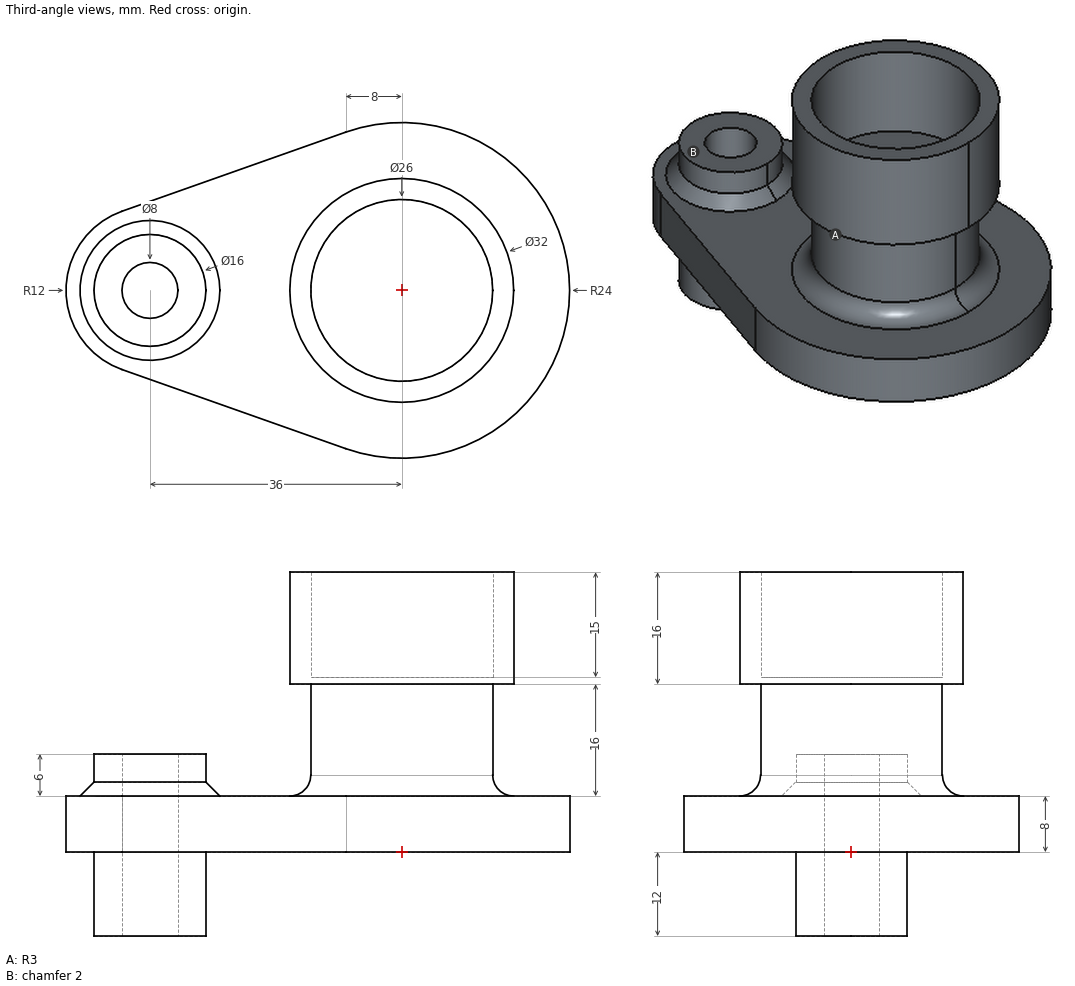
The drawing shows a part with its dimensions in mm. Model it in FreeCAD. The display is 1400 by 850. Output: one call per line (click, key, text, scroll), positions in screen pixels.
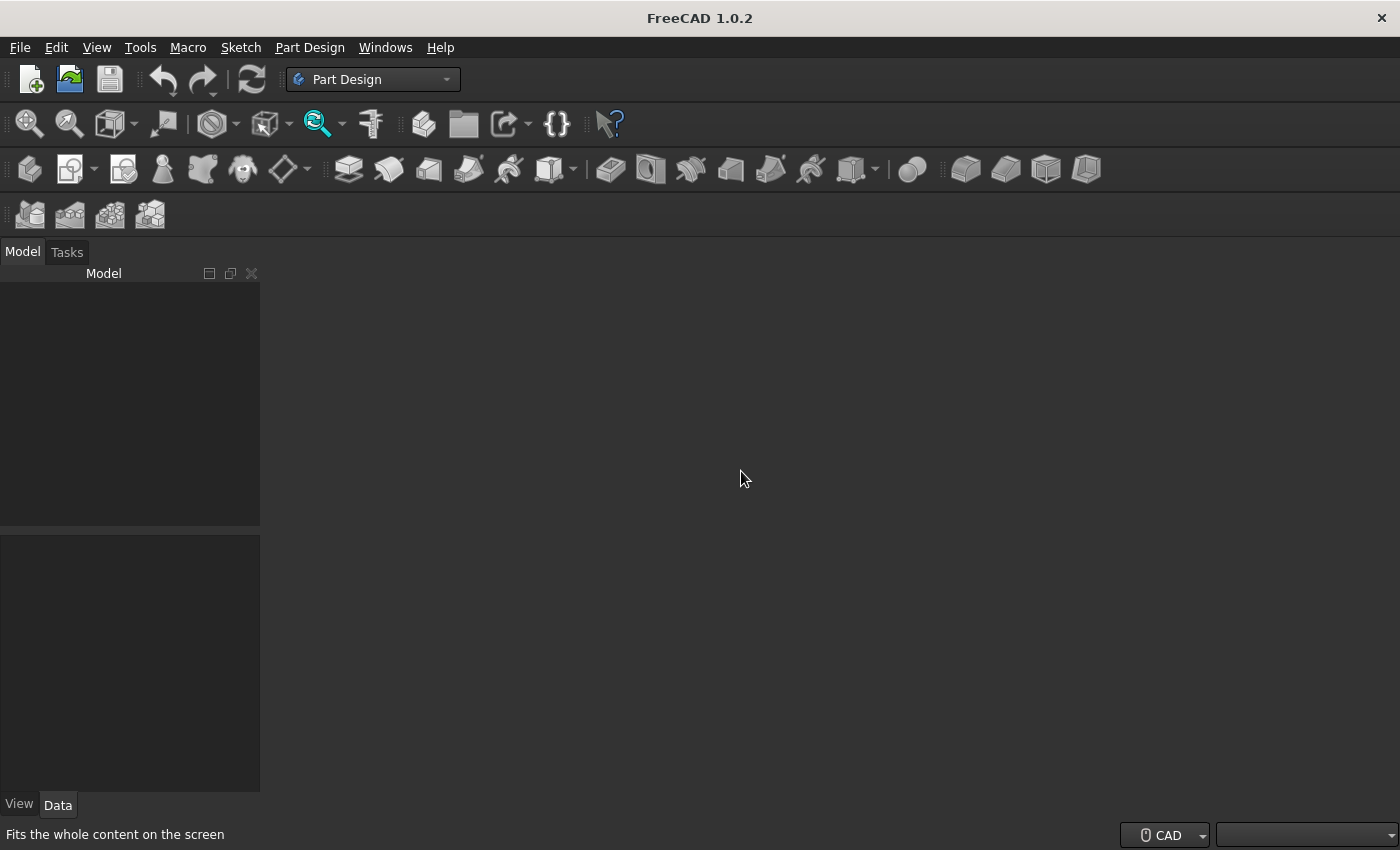
key(ctrl+n)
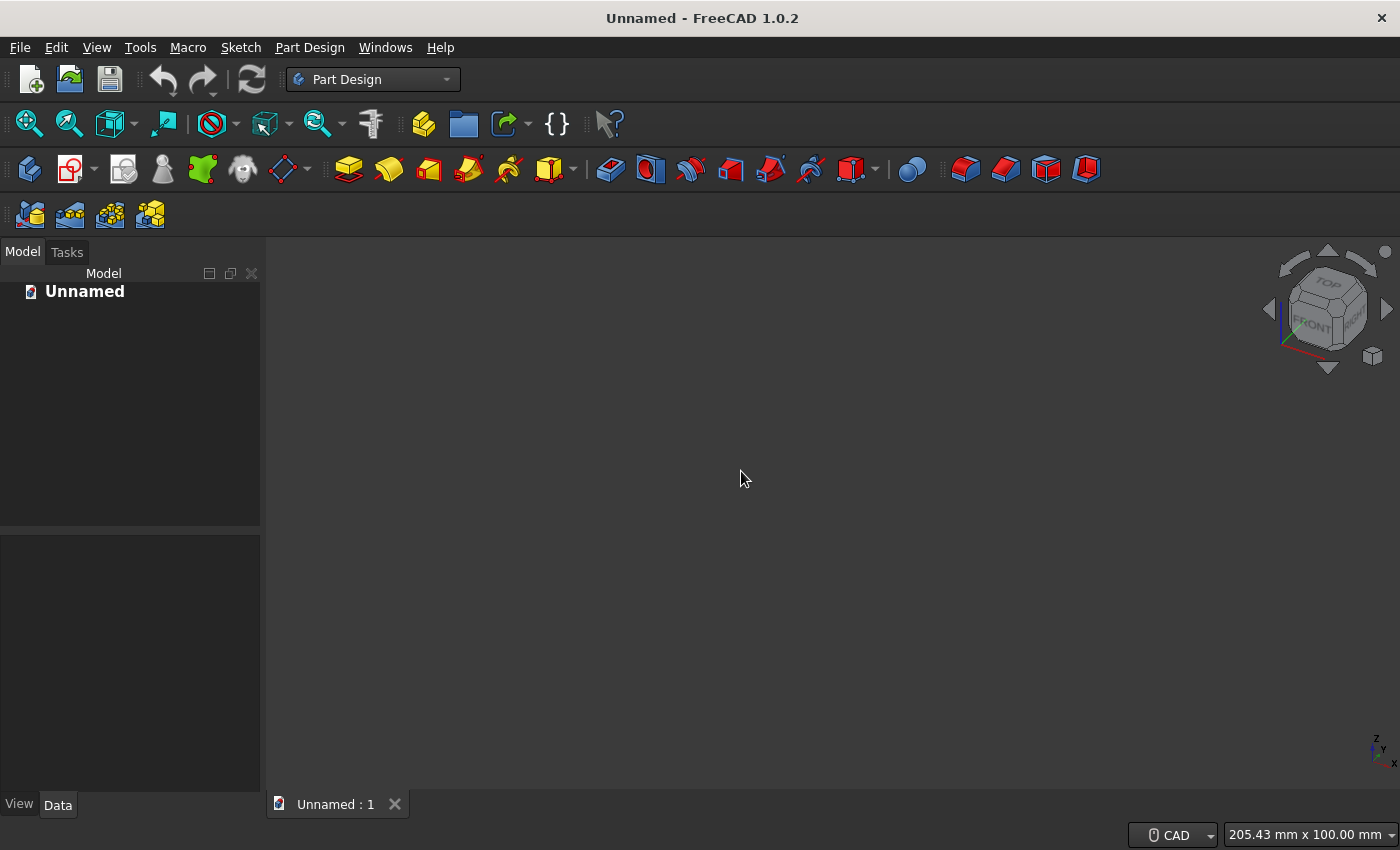
click(70, 170)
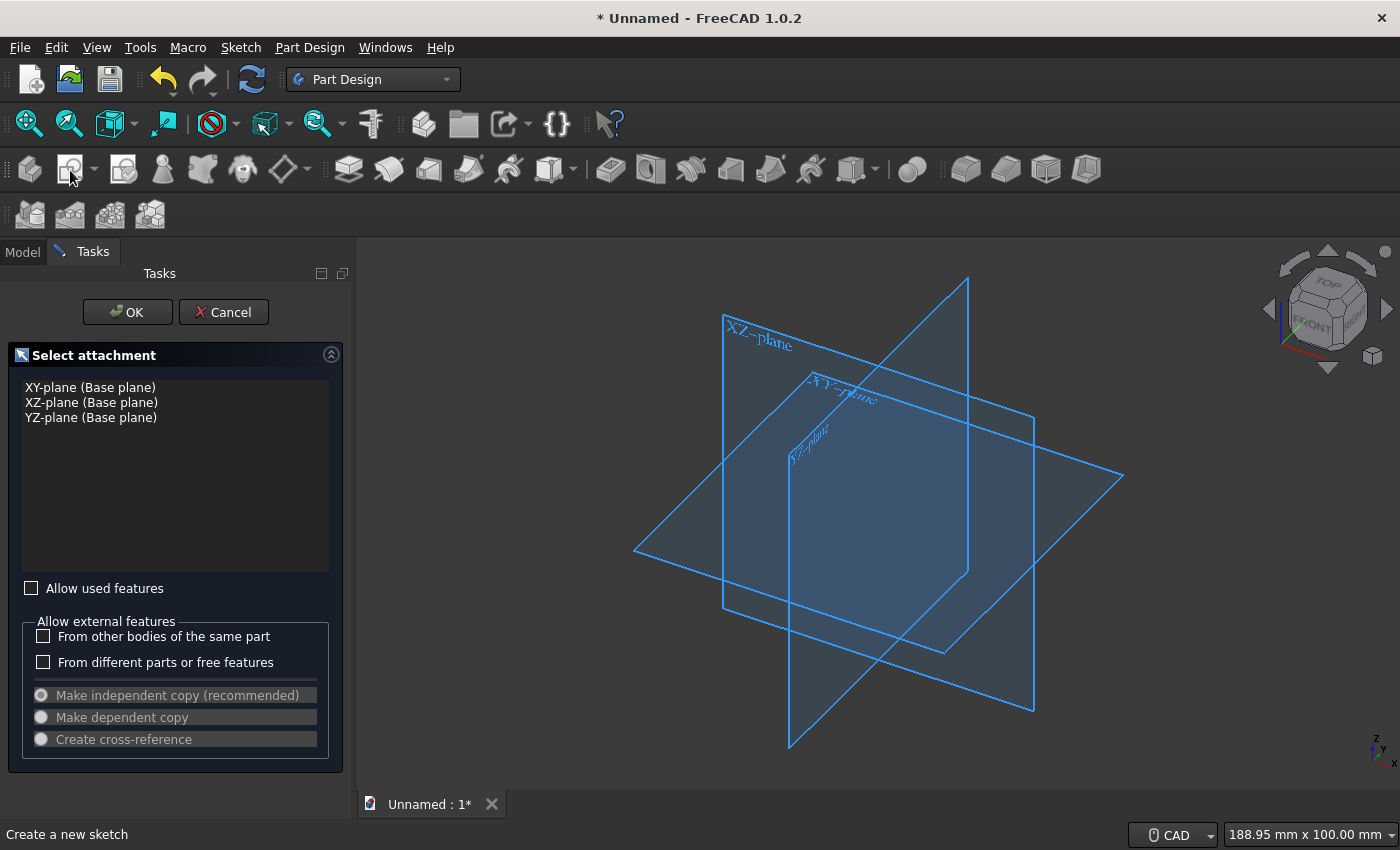
click(82, 388)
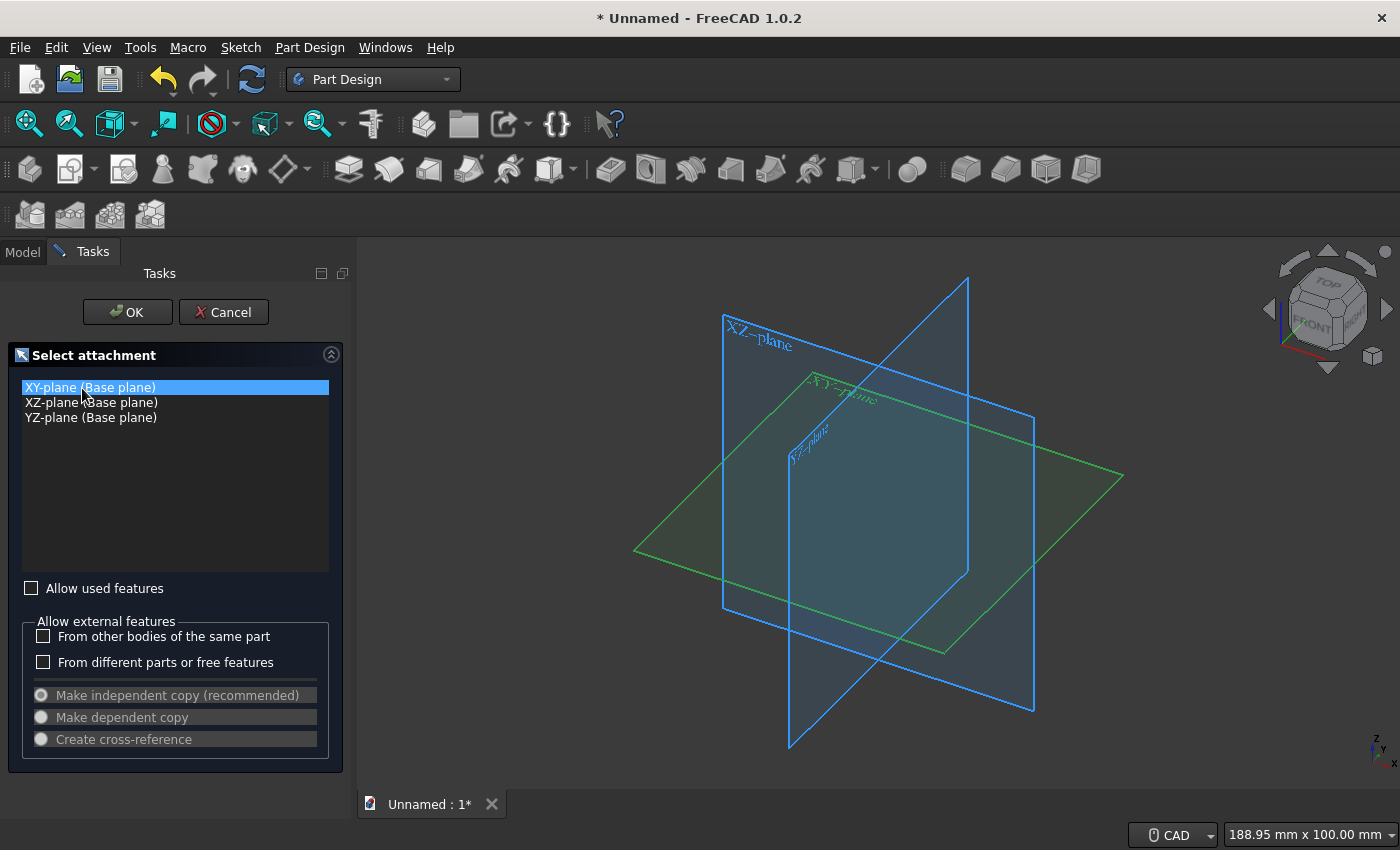
click(128, 312)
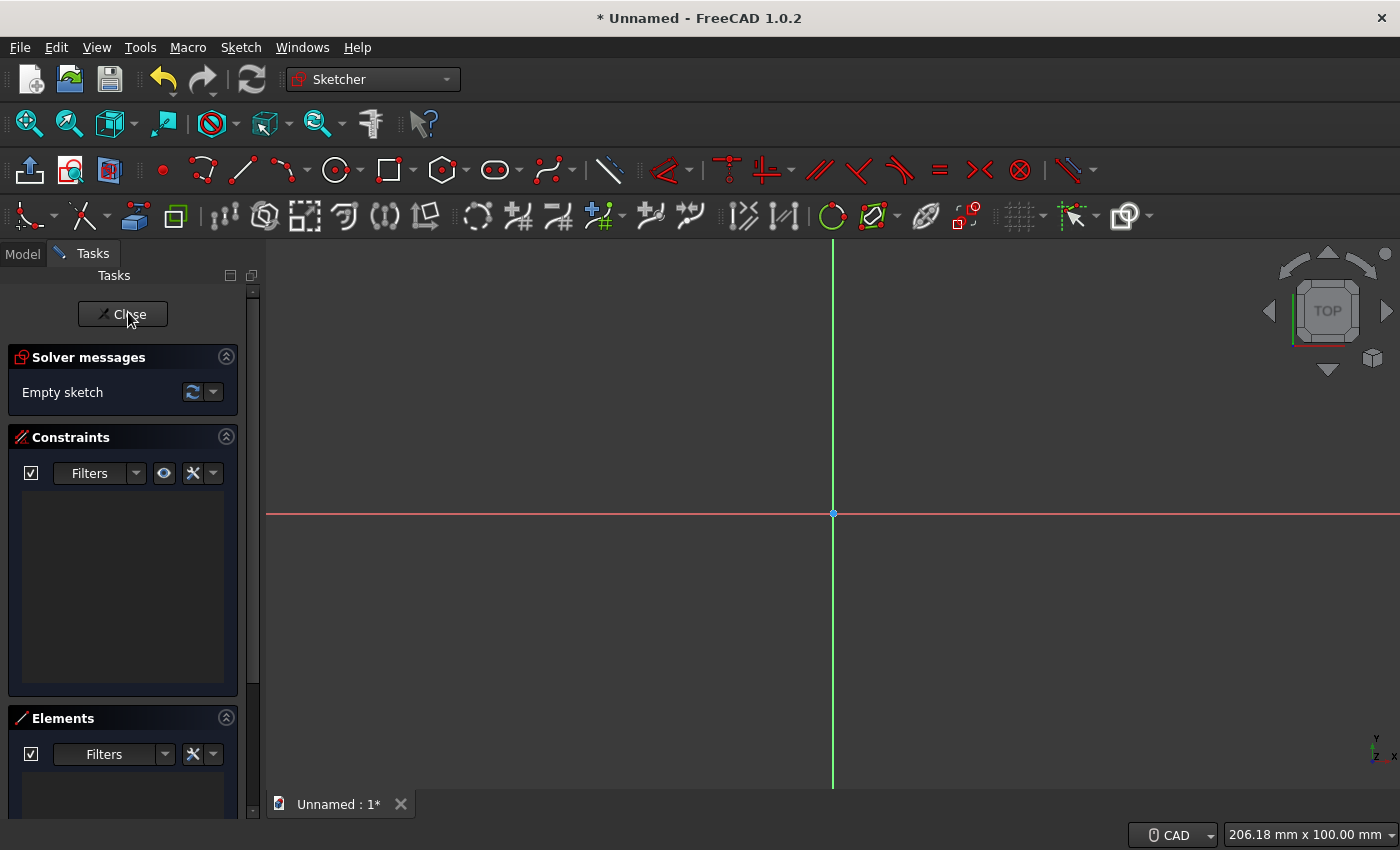
scroll(772, 514, up, 2)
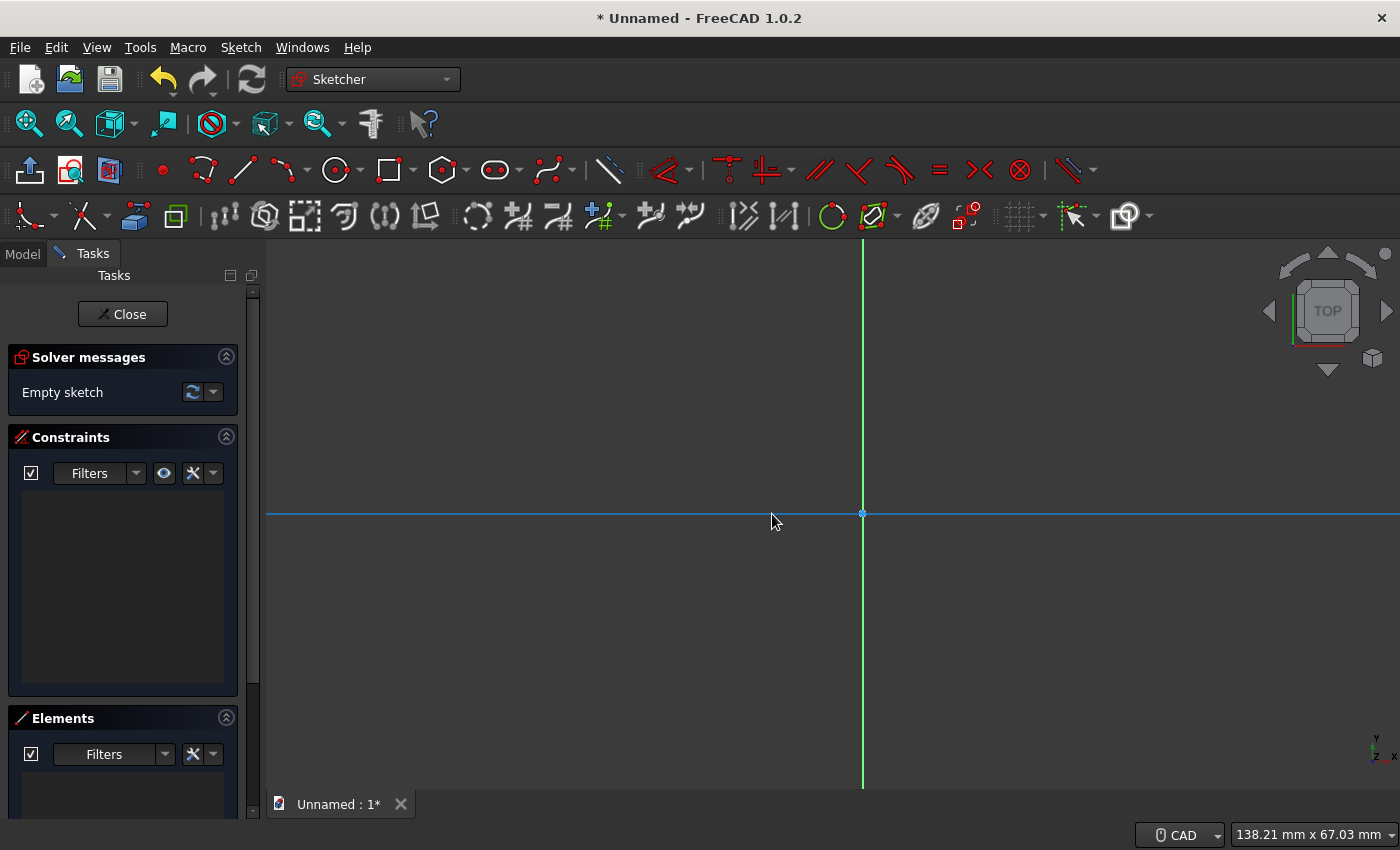
key(g)
key(l)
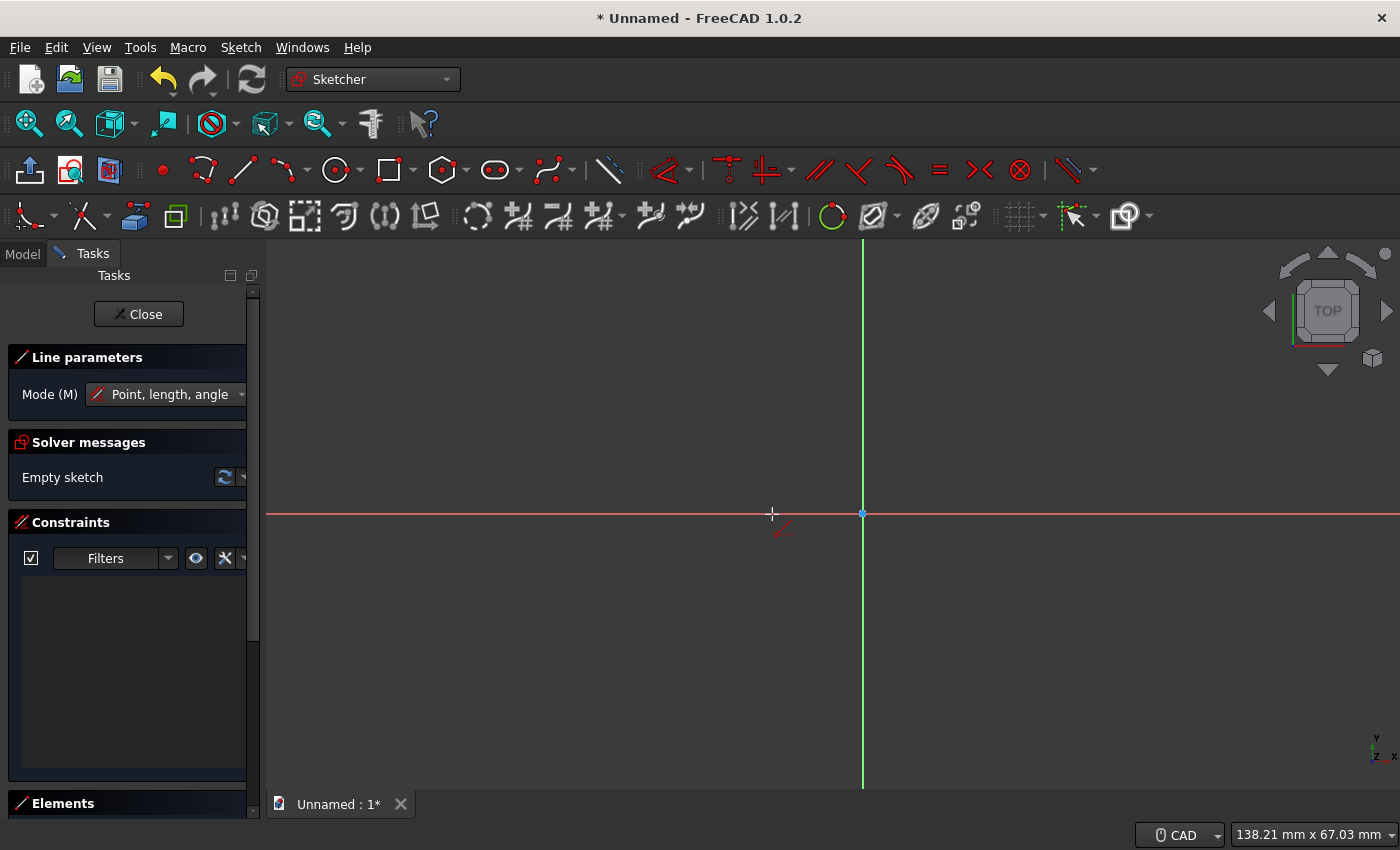
click(797, 328)
click(535, 421)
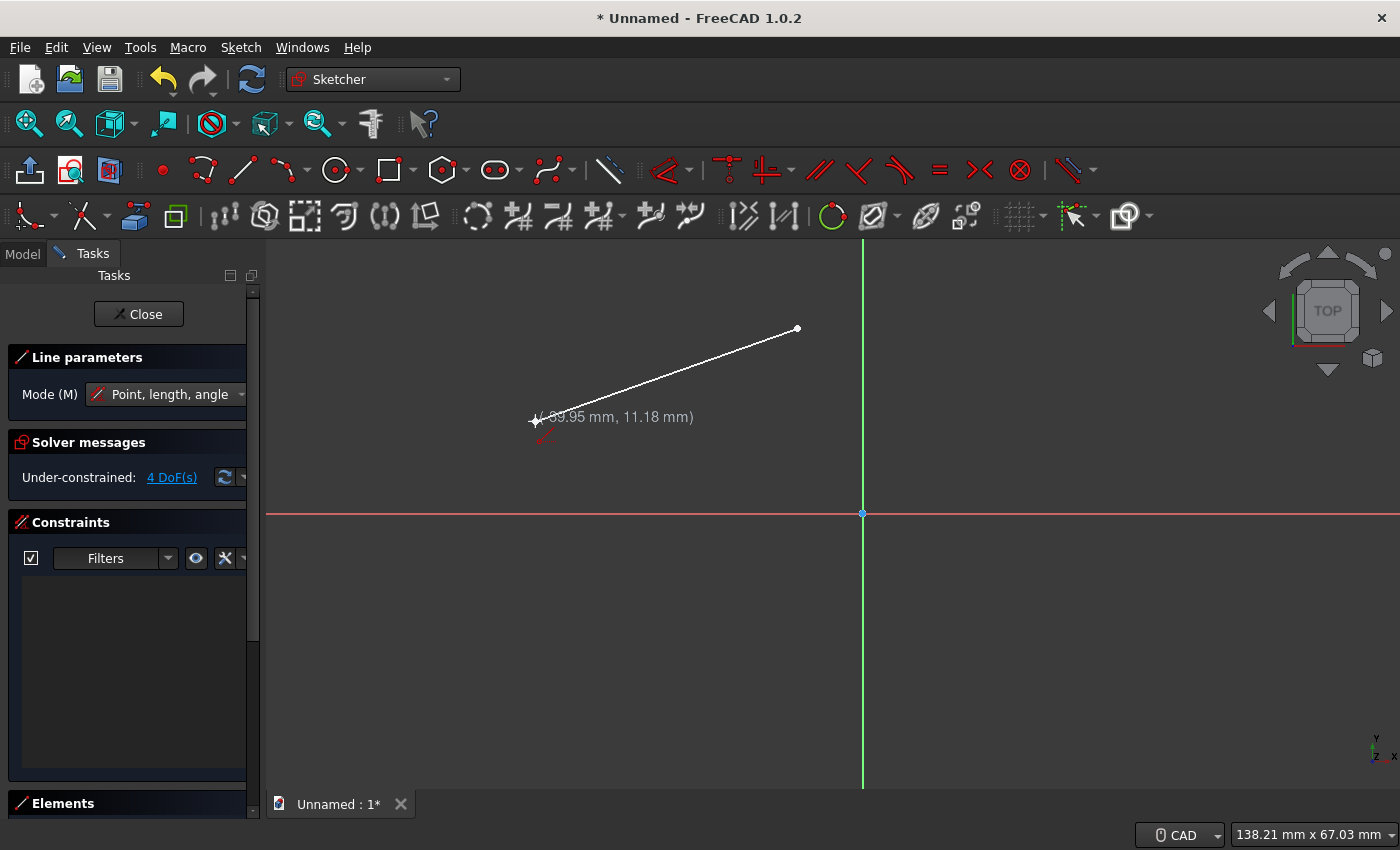
click(535, 607)
click(797, 699)